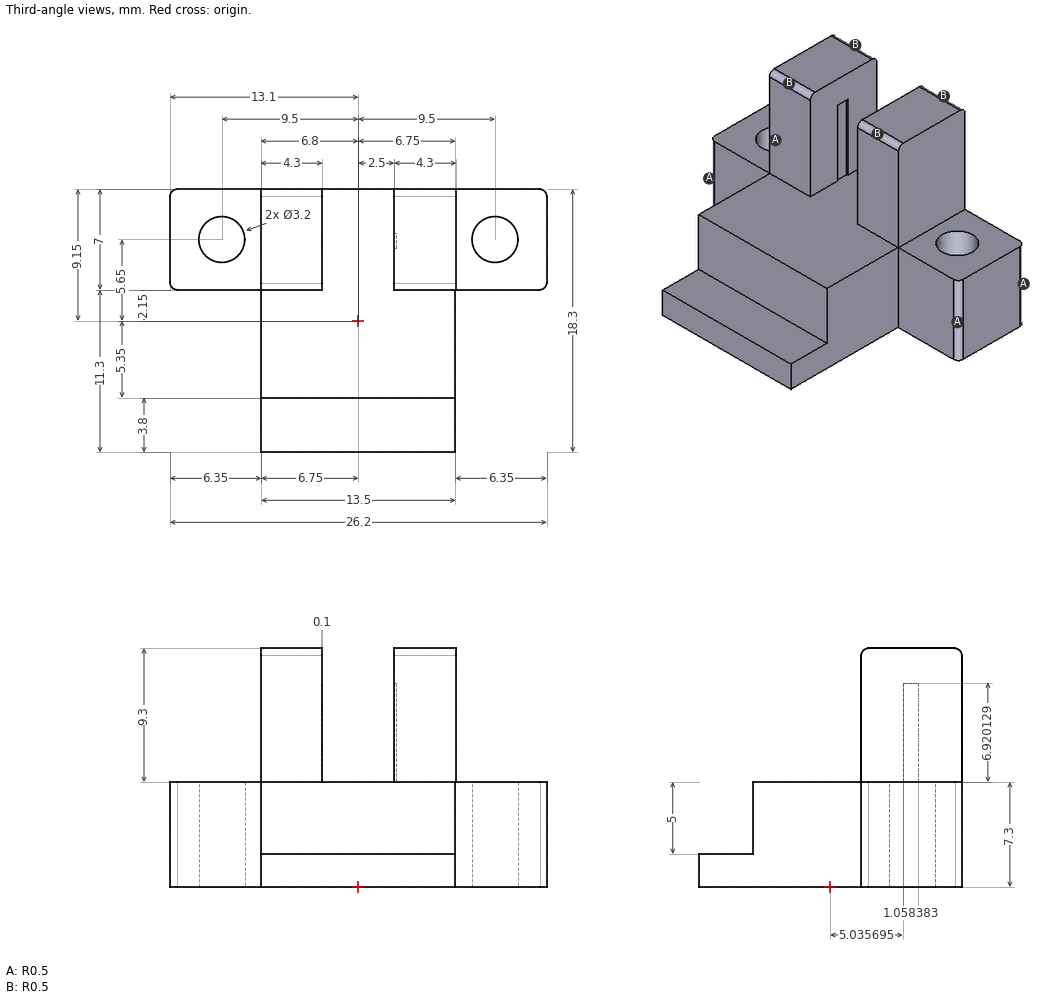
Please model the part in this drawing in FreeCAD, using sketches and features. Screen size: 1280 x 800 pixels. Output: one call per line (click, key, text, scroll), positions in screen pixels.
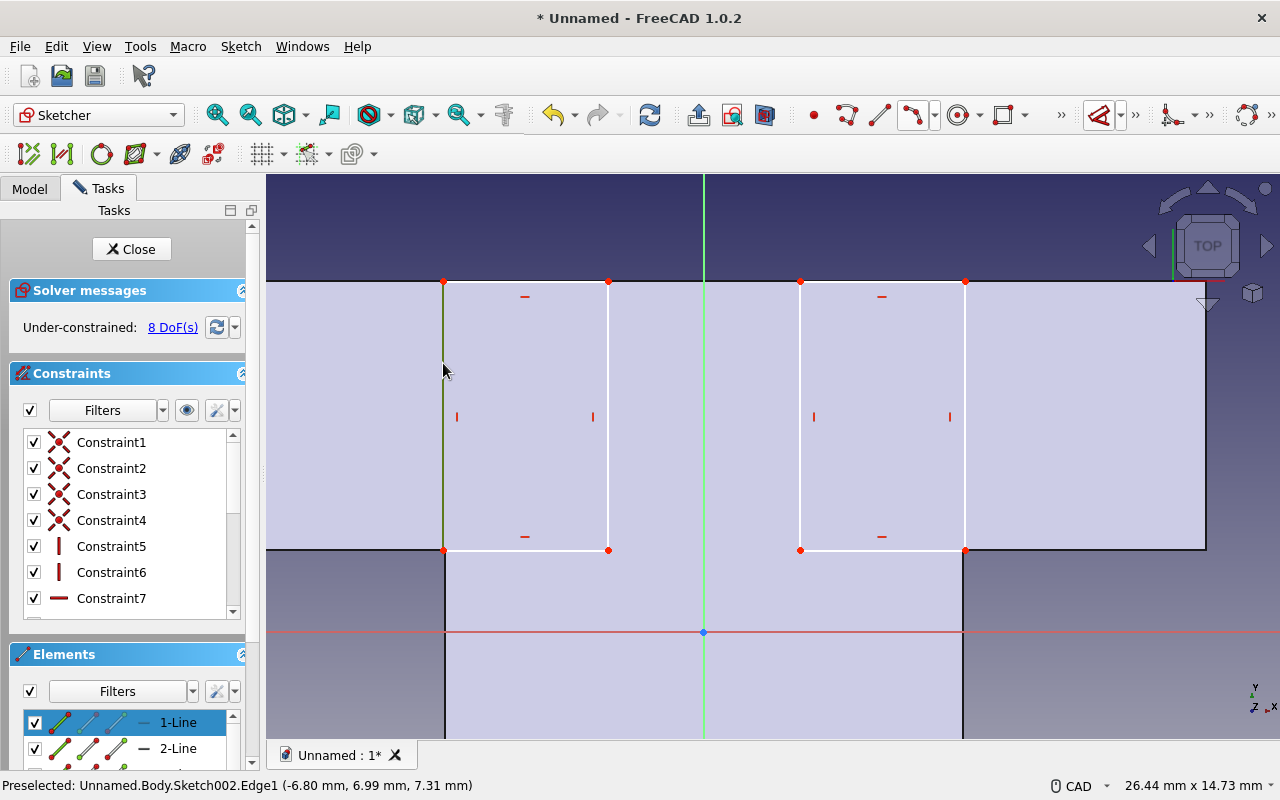
key(i)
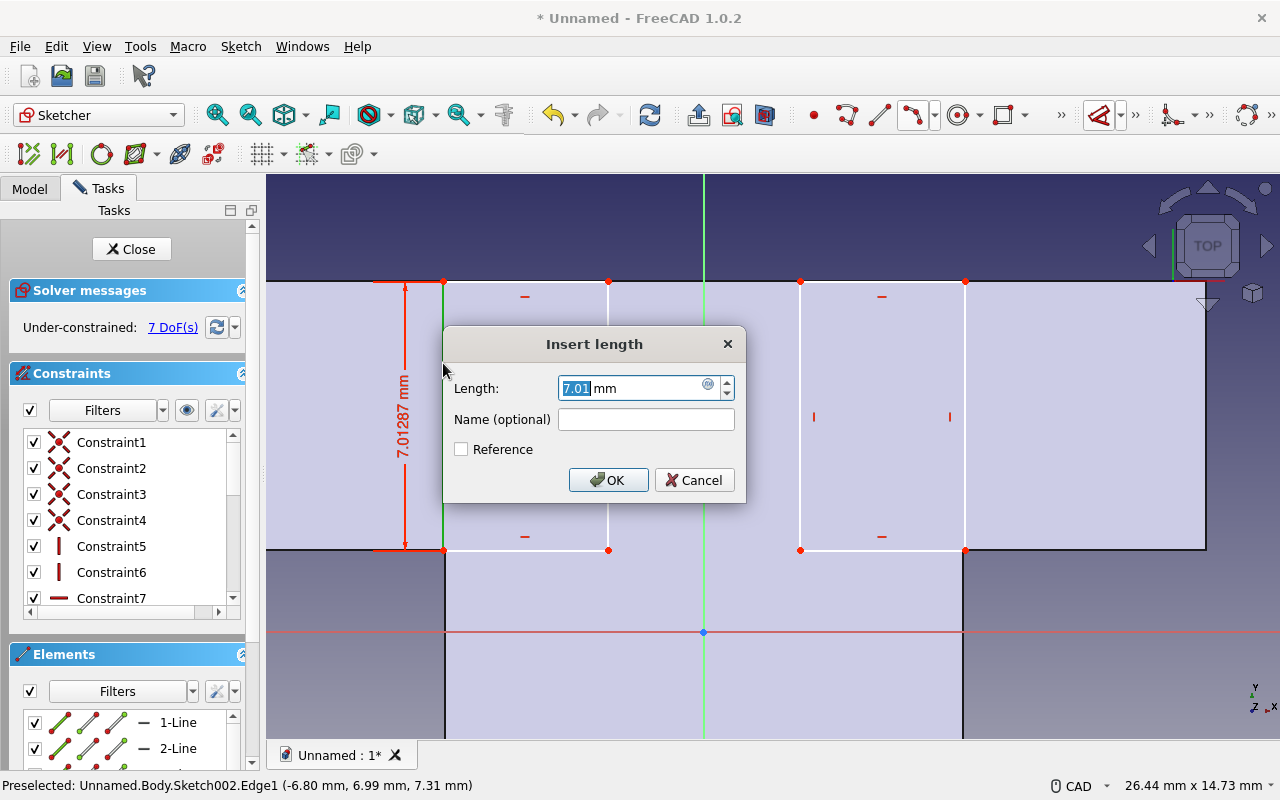
text(7)
key(Return)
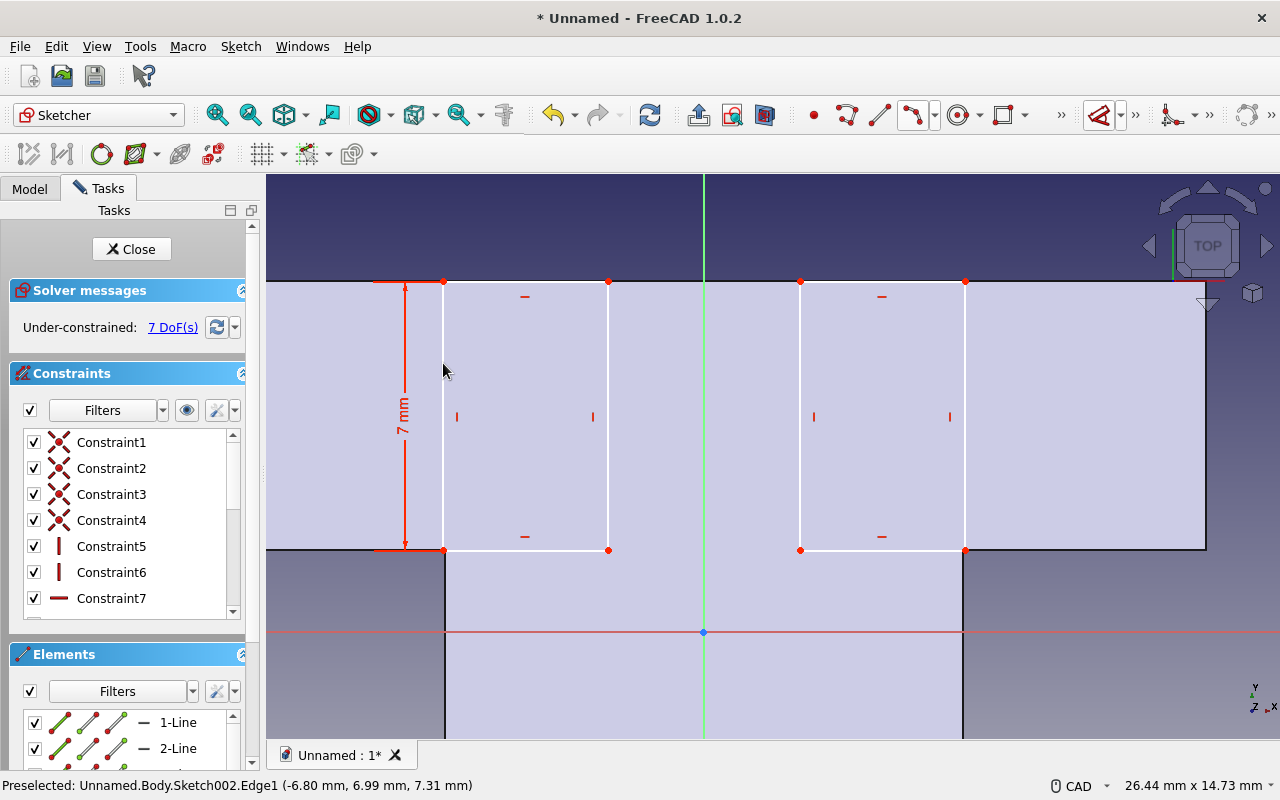
click(800, 363)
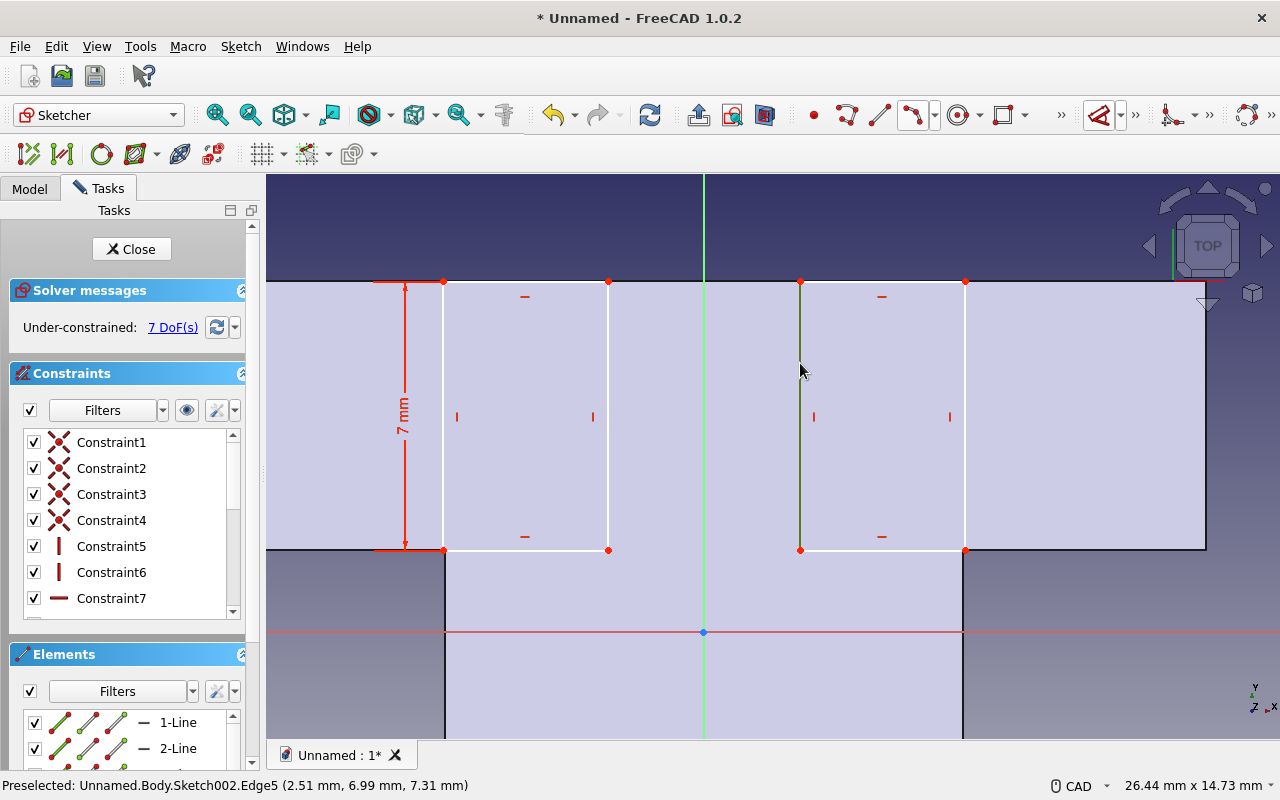
key(i)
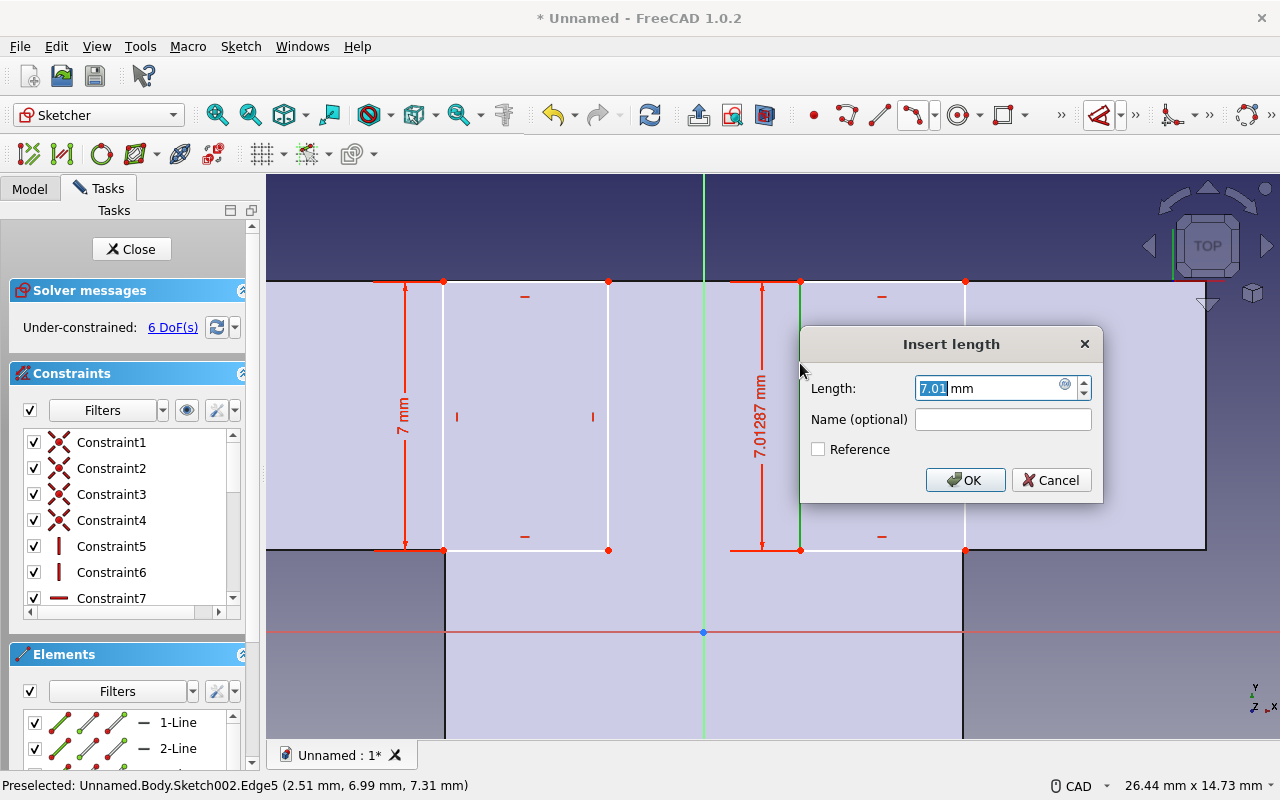
text(7)
key(Return)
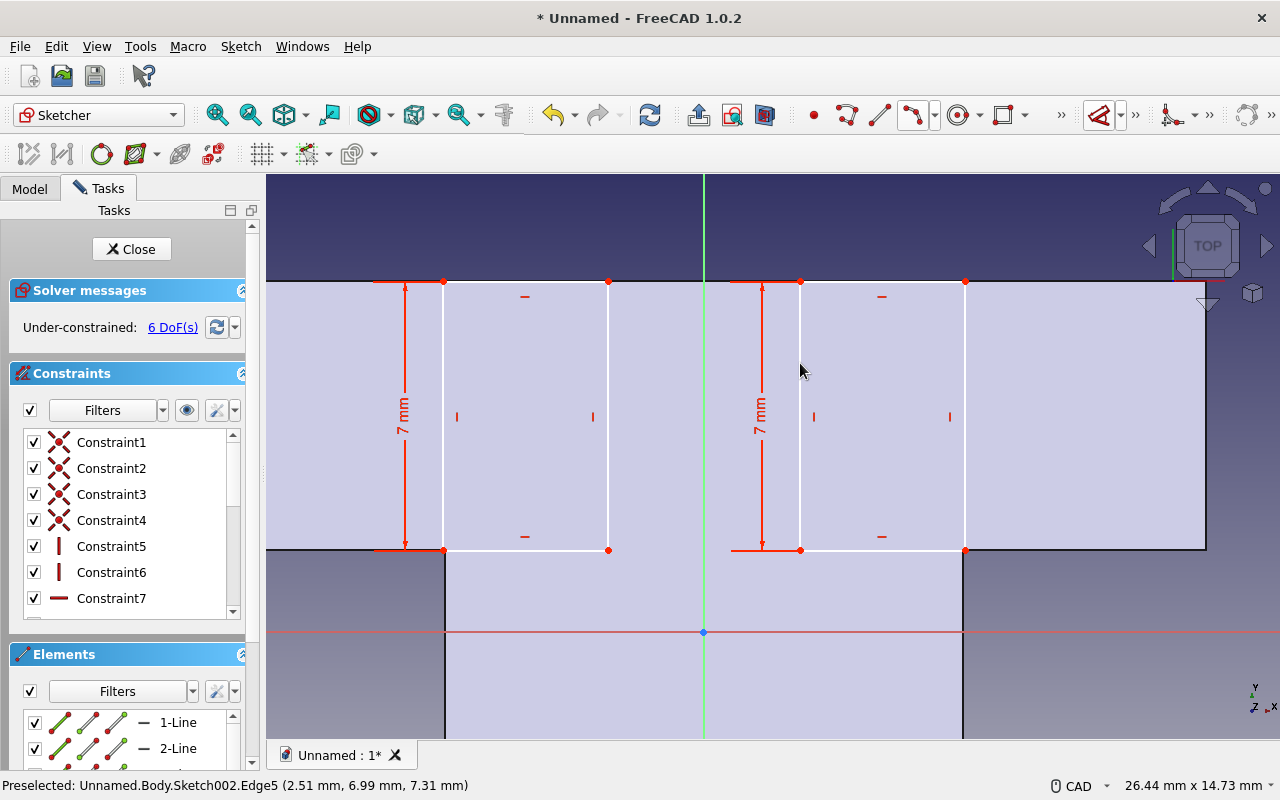
click(492, 551)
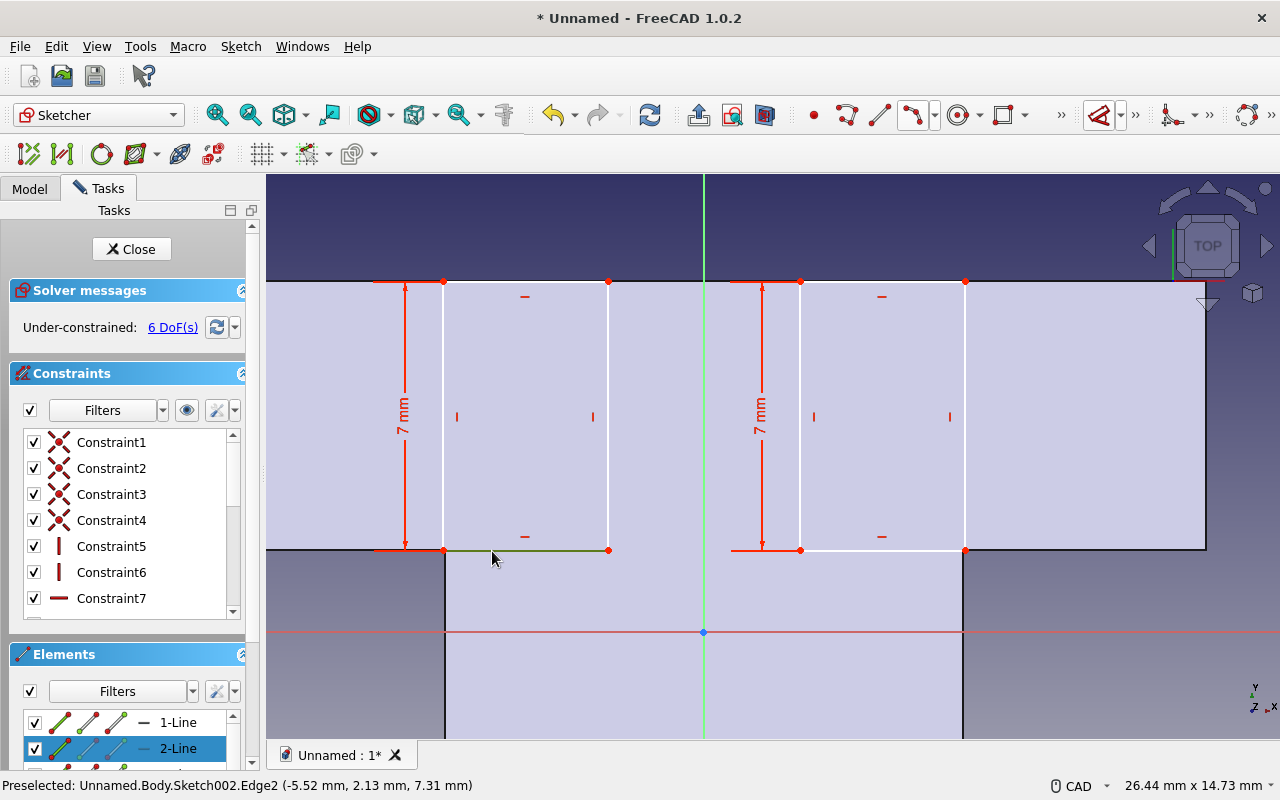
key(l)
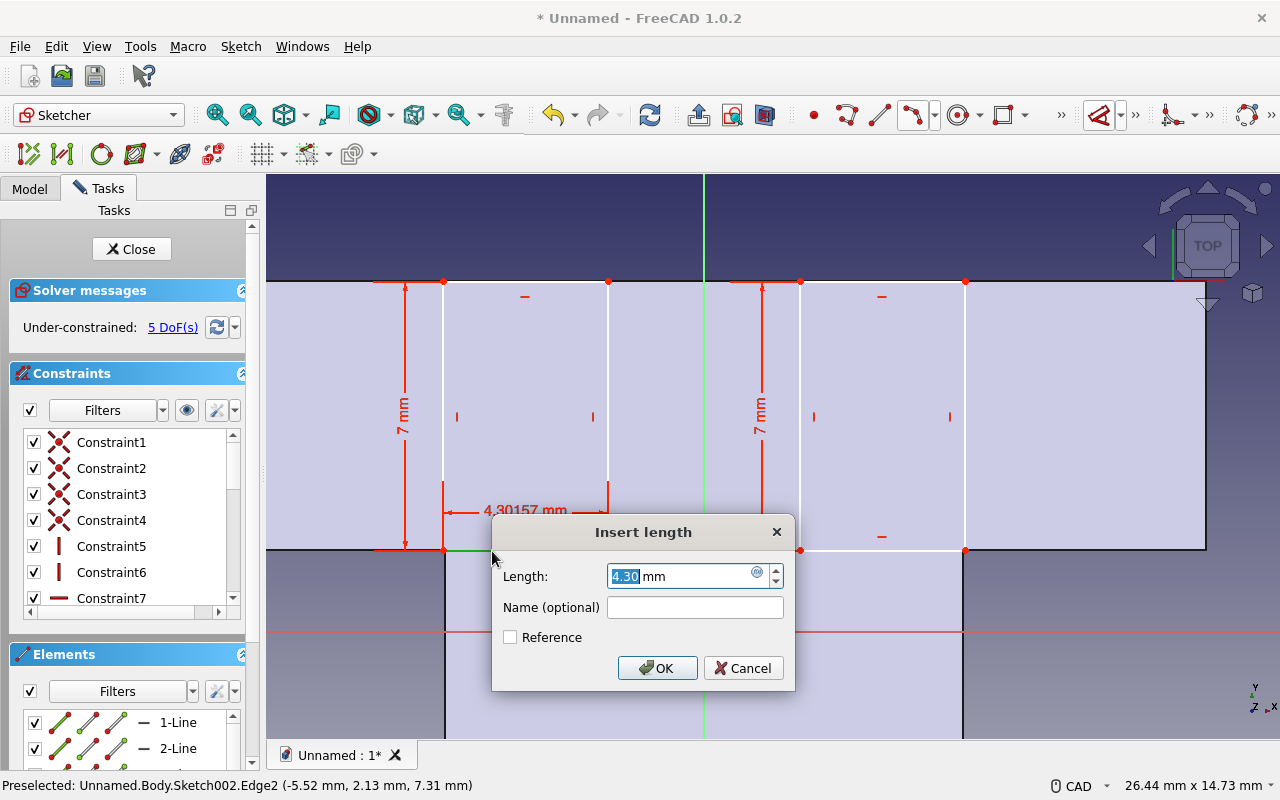
text(4.3)
key(Return)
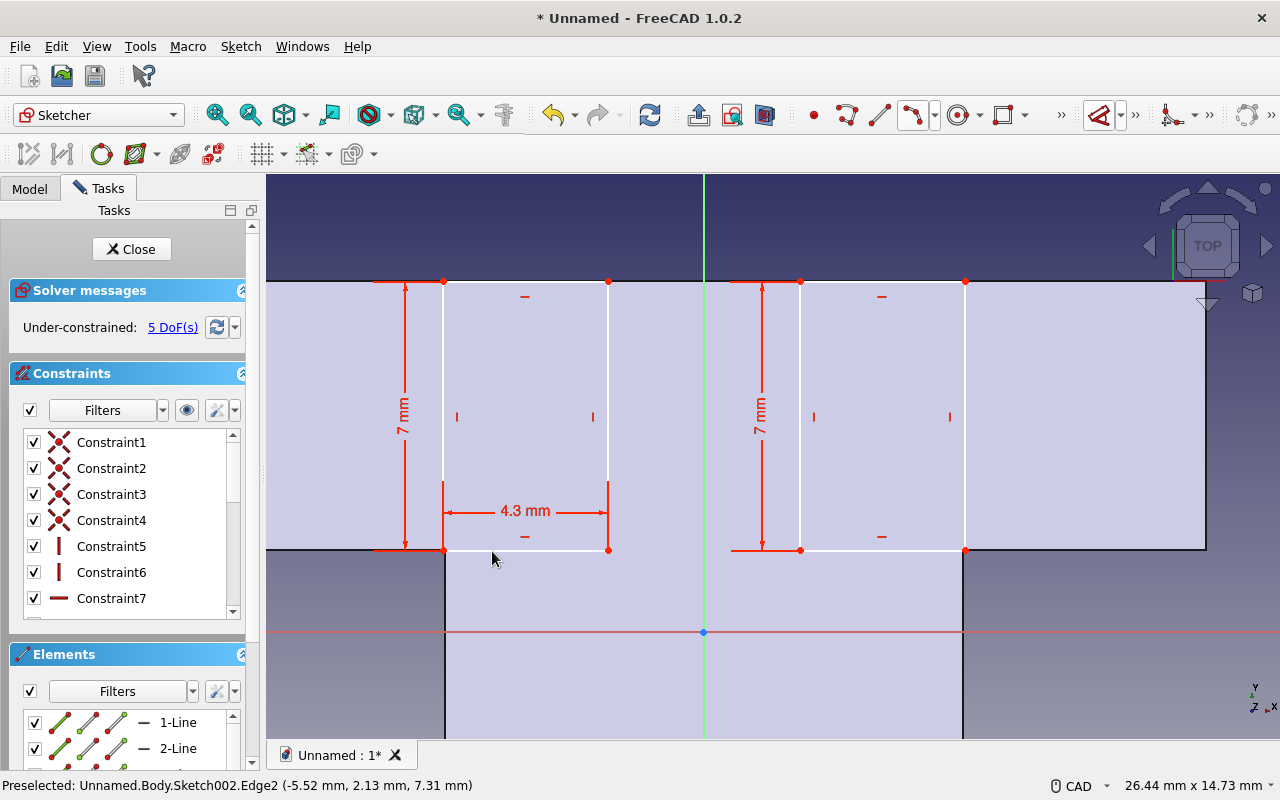
click(850, 551)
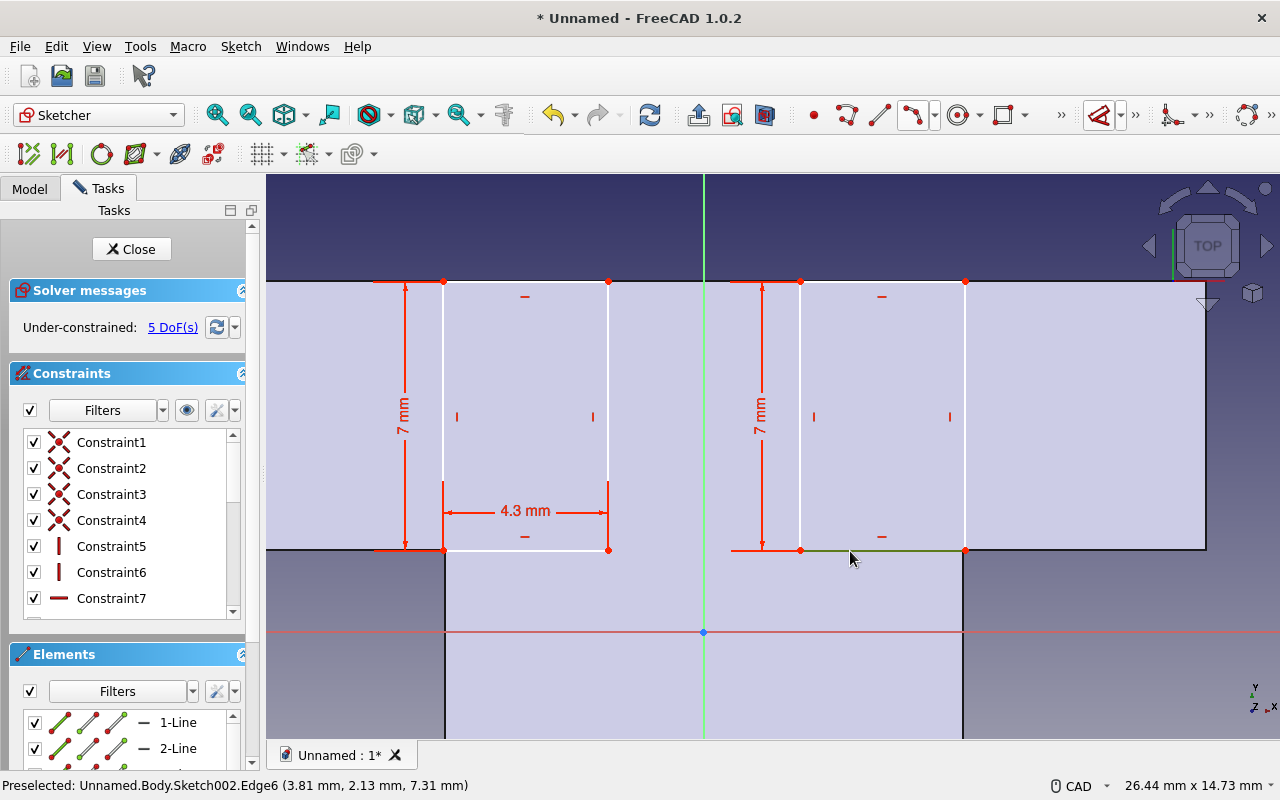
key(l)